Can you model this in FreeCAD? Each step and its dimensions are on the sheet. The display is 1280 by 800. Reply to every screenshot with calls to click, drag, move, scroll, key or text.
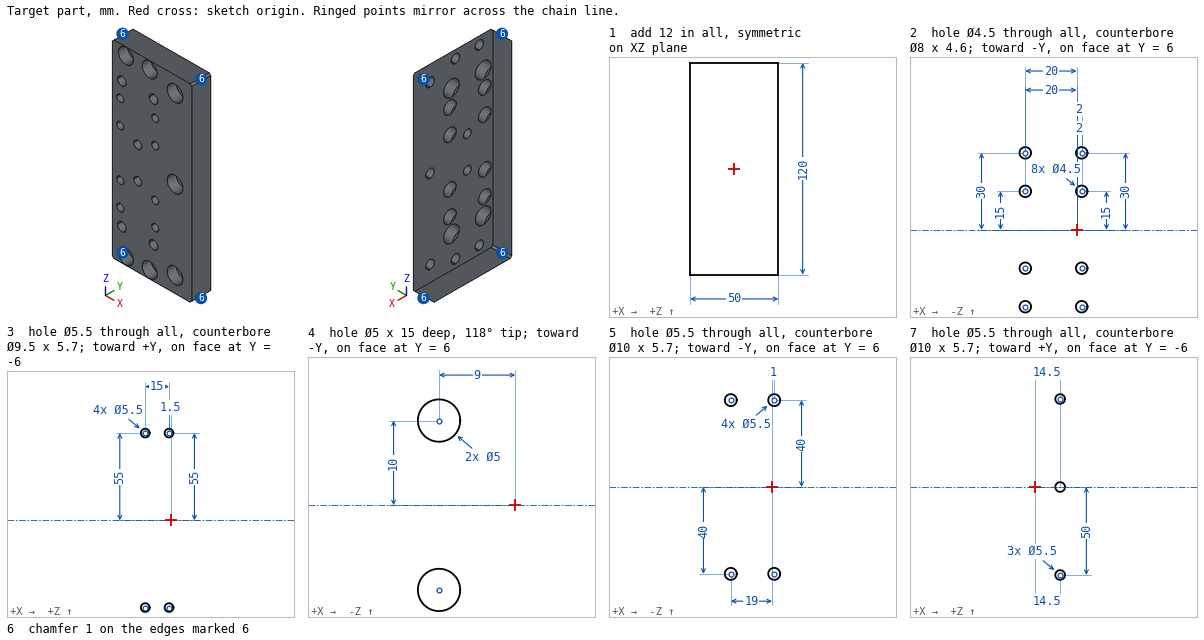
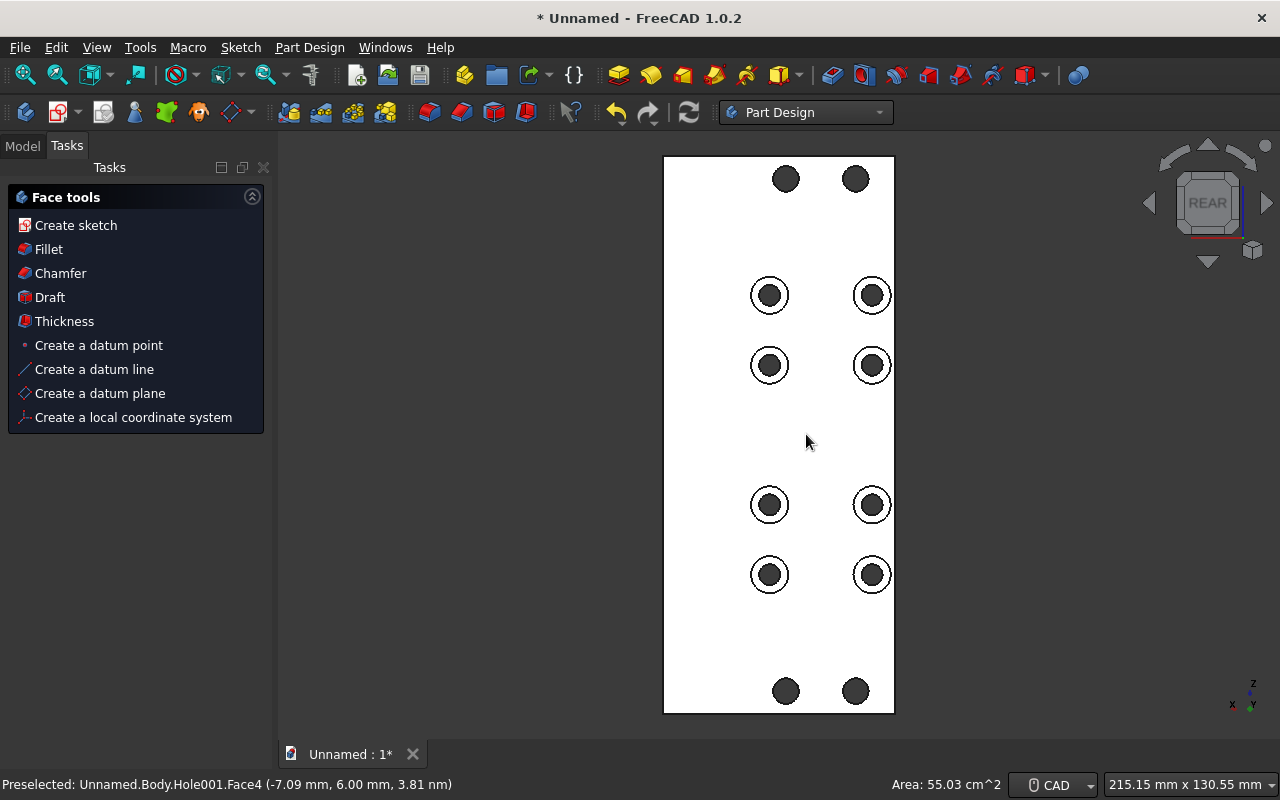
click(58, 112)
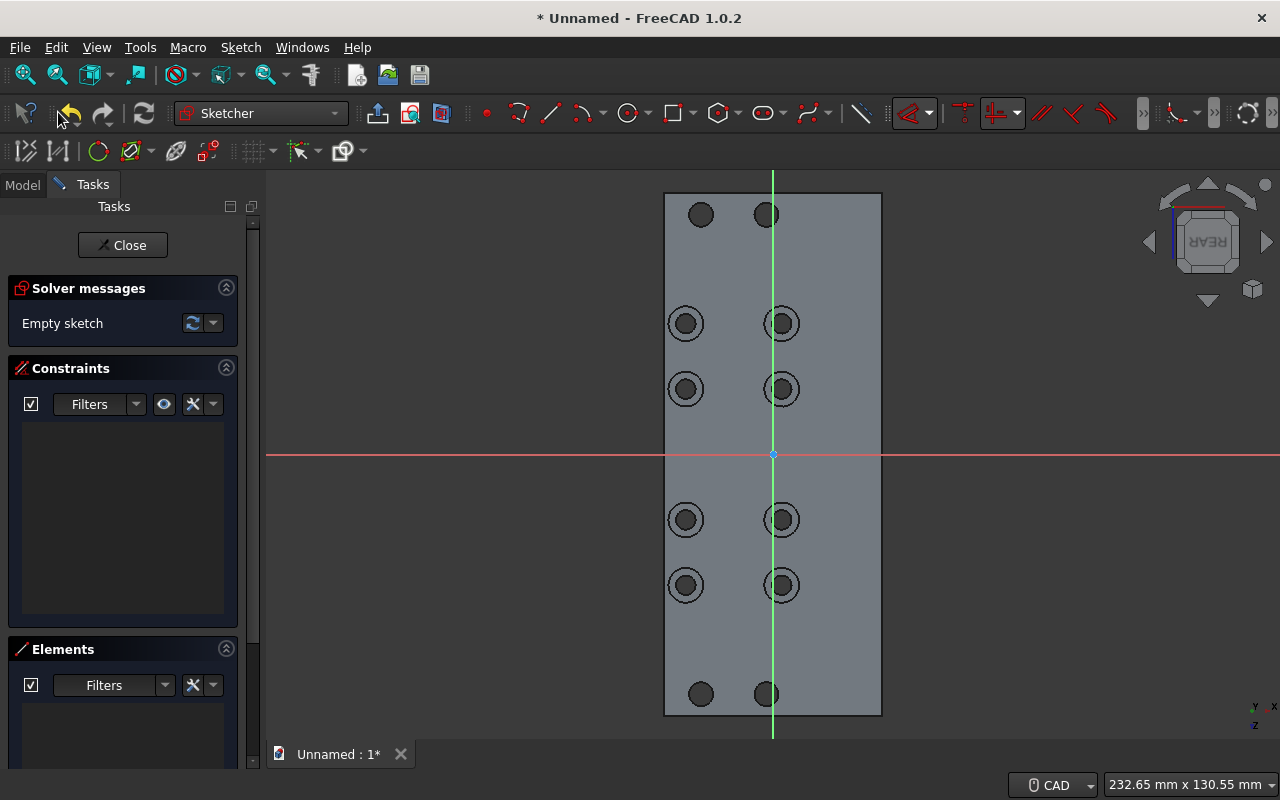
scroll(767, 455, up, 6)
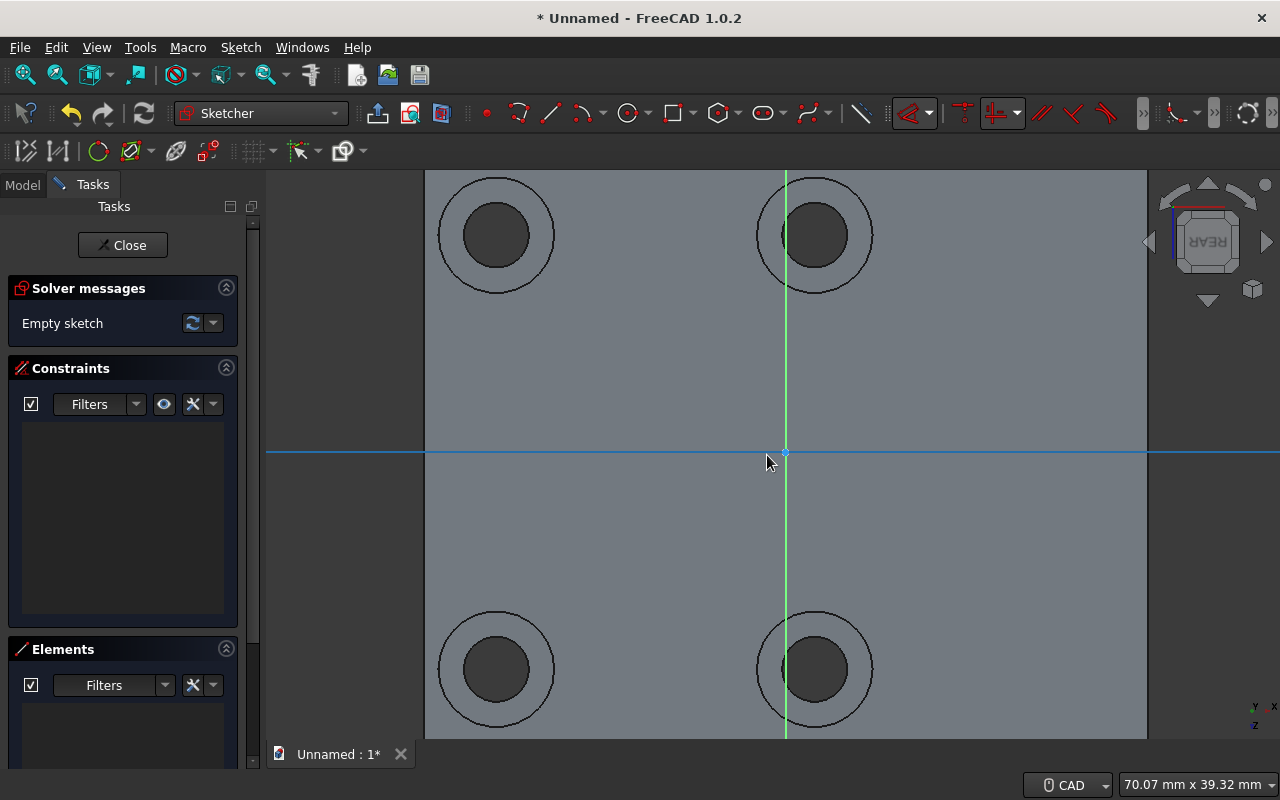
click(628, 114)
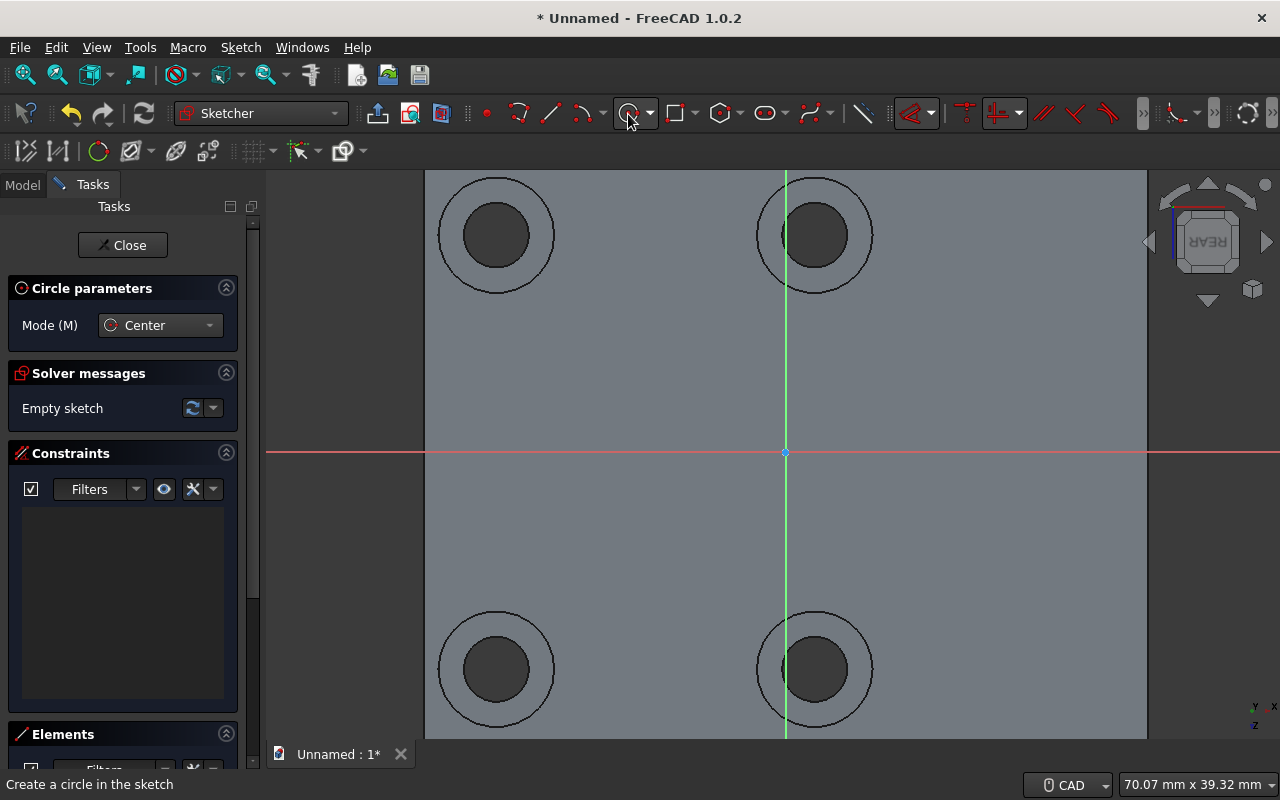
click(656, 307)
move(681, 282)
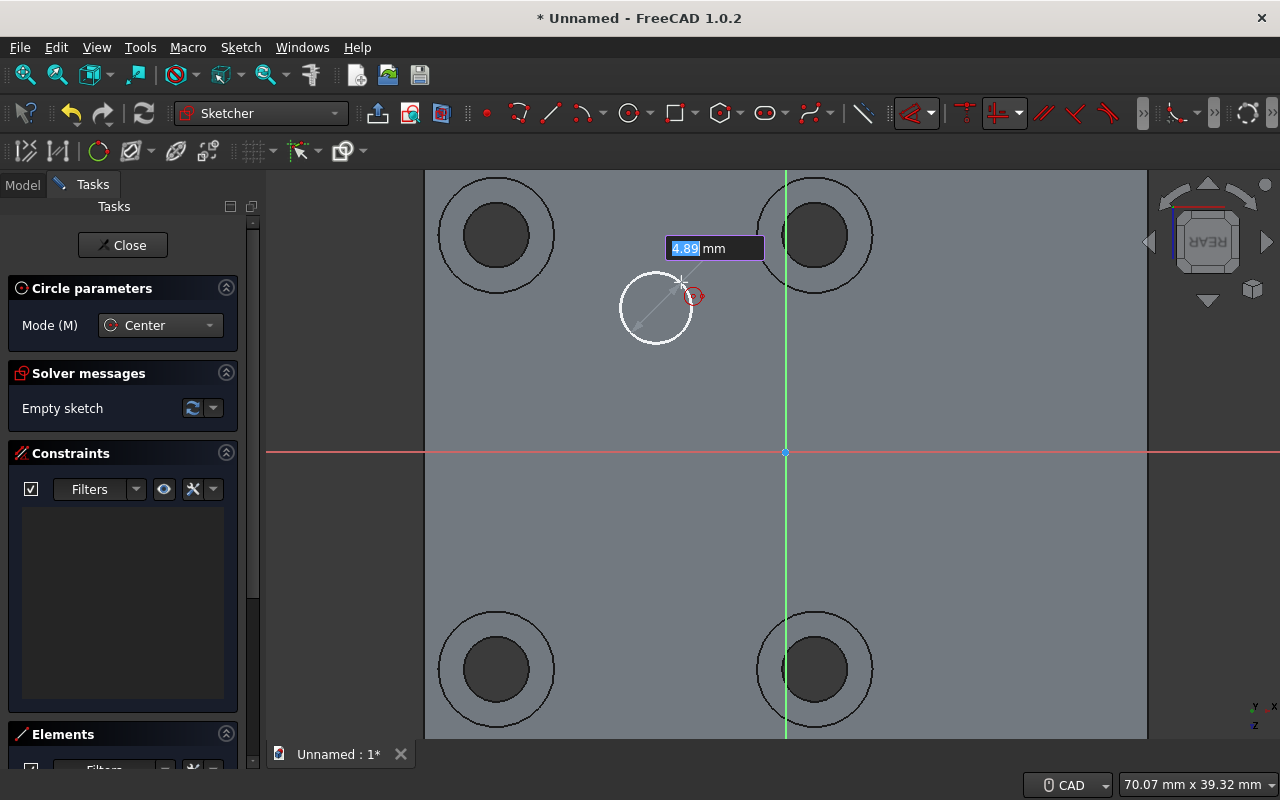
text(5)
key(Return)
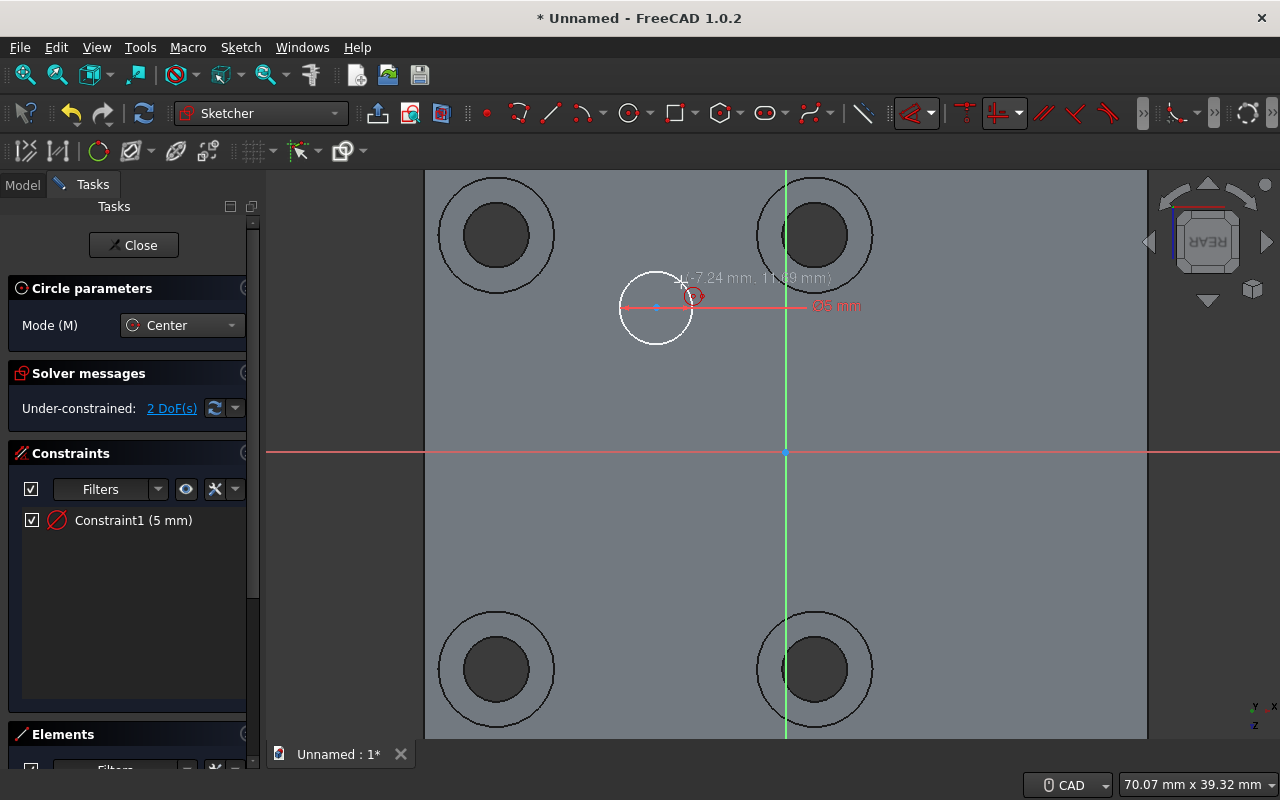
click(656, 597)
move(681, 571)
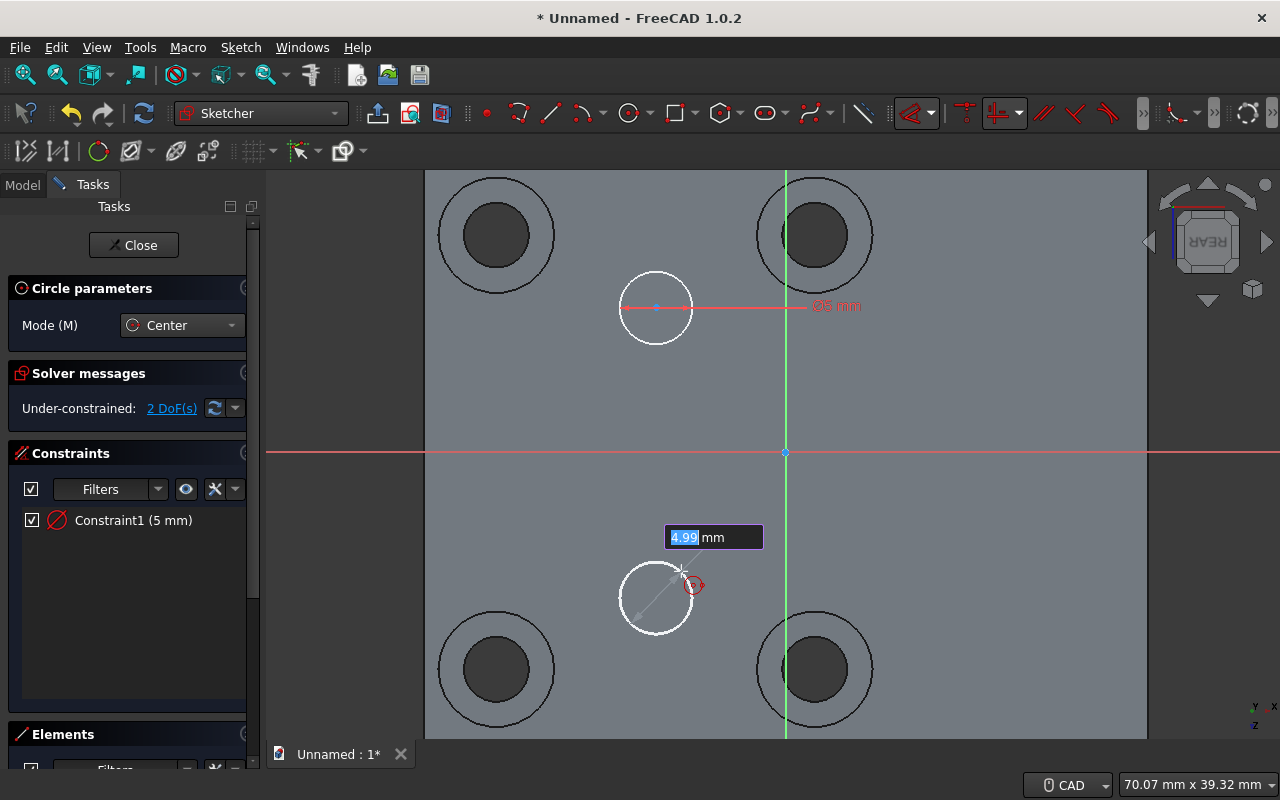
text(5)
key(Return)
key(Escape)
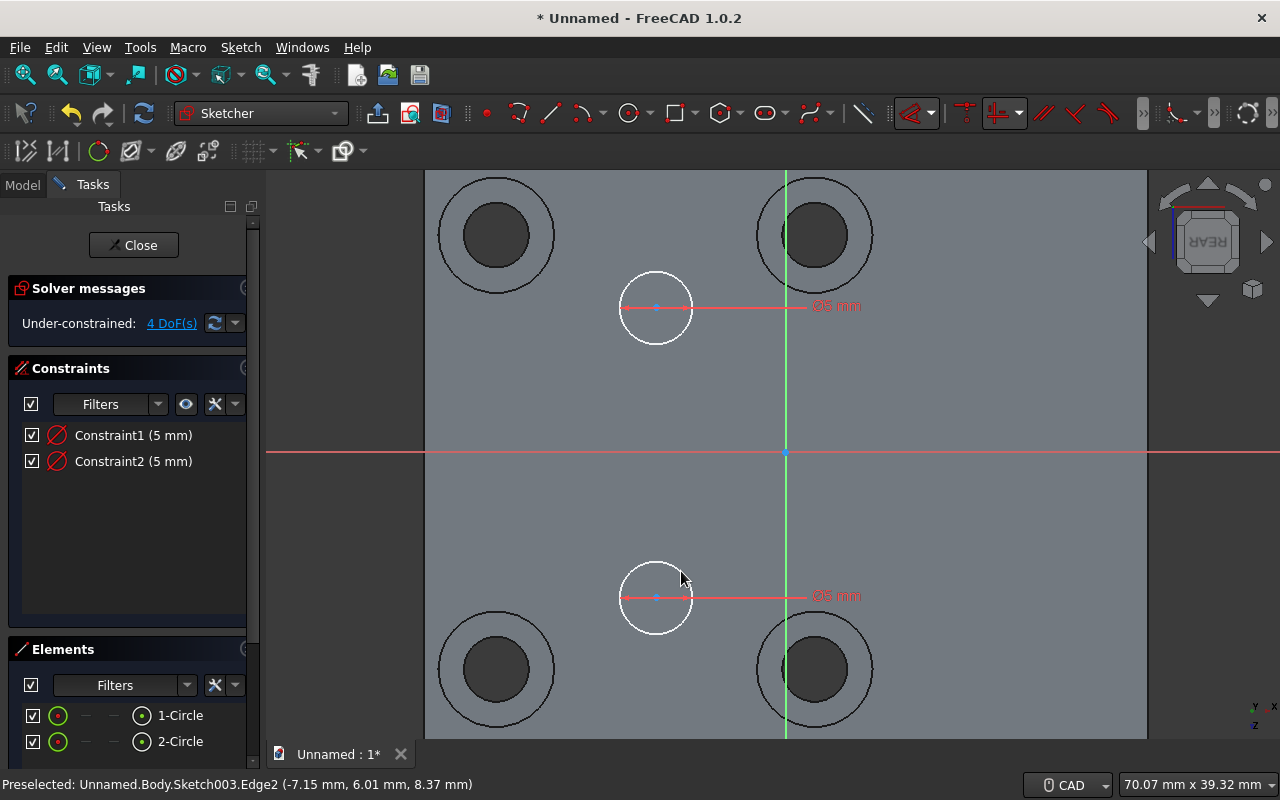
click(656, 308)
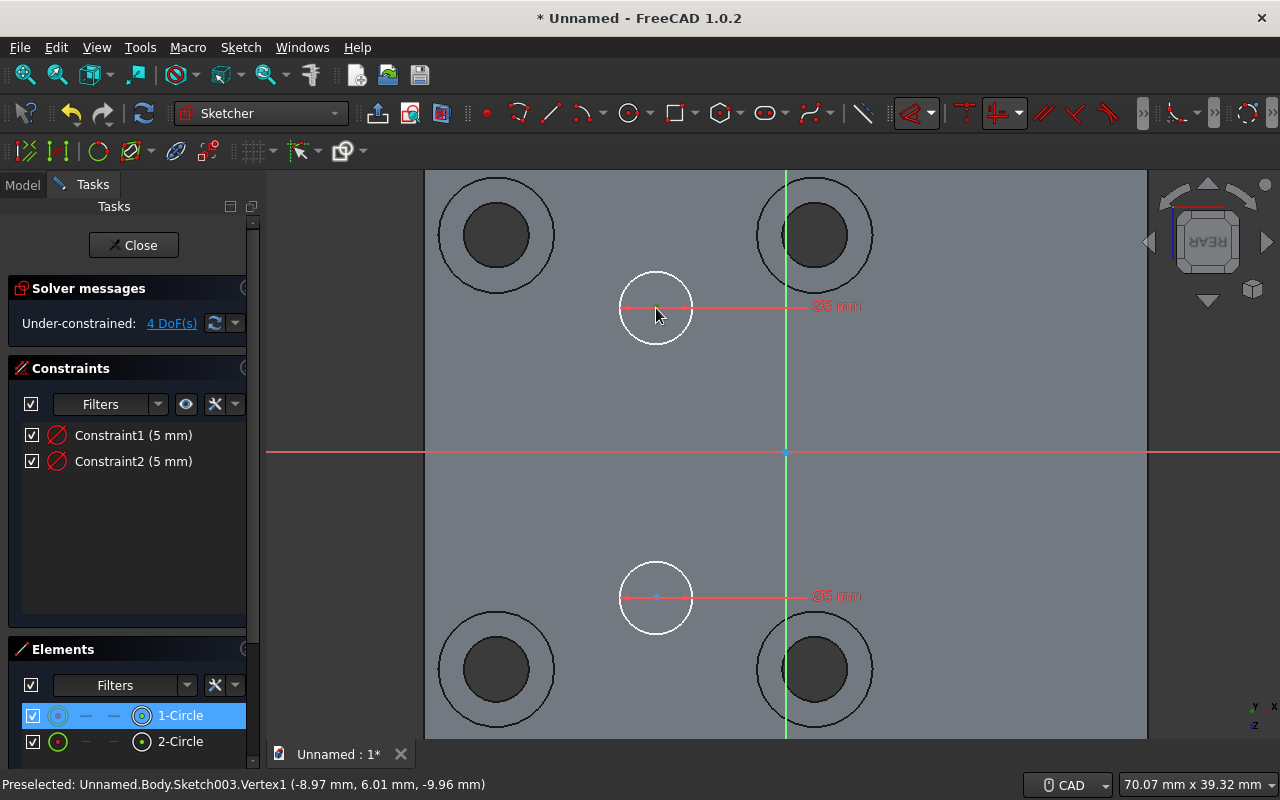
click(656, 598)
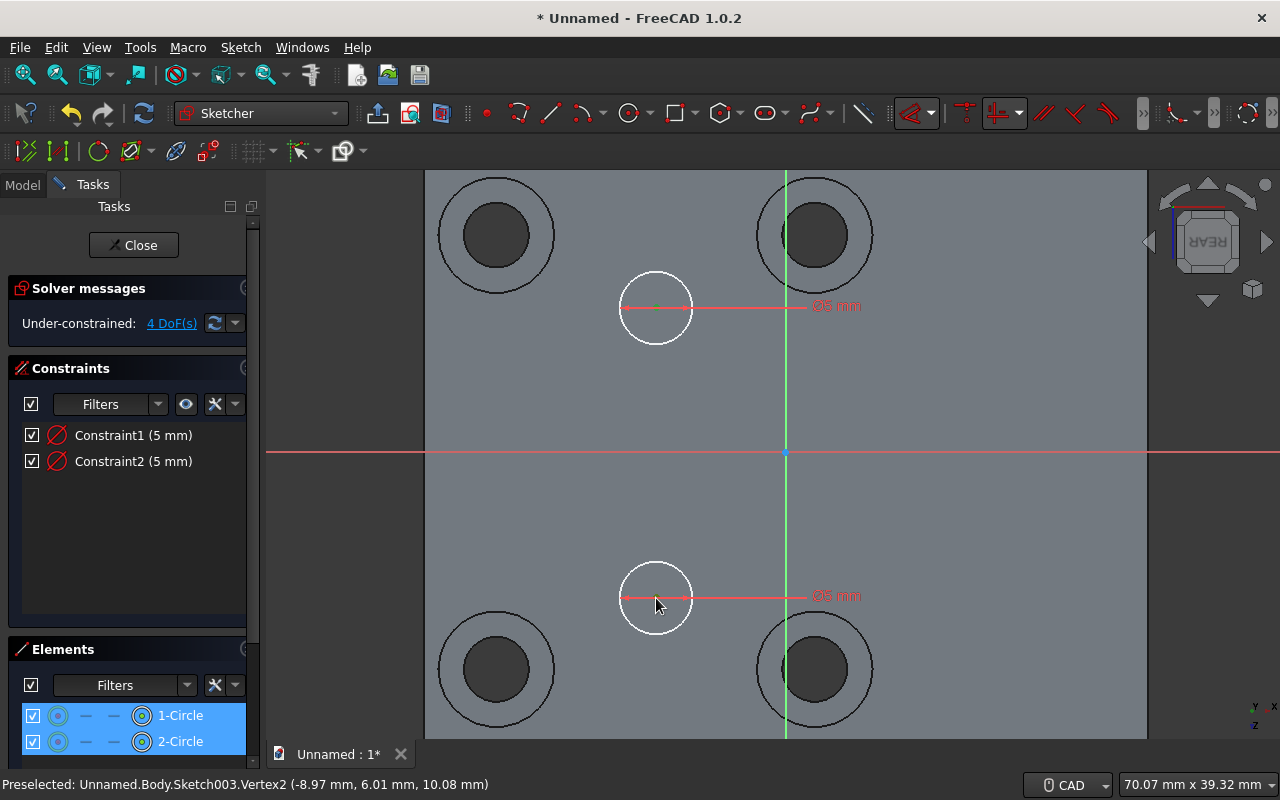
click(353, 452)